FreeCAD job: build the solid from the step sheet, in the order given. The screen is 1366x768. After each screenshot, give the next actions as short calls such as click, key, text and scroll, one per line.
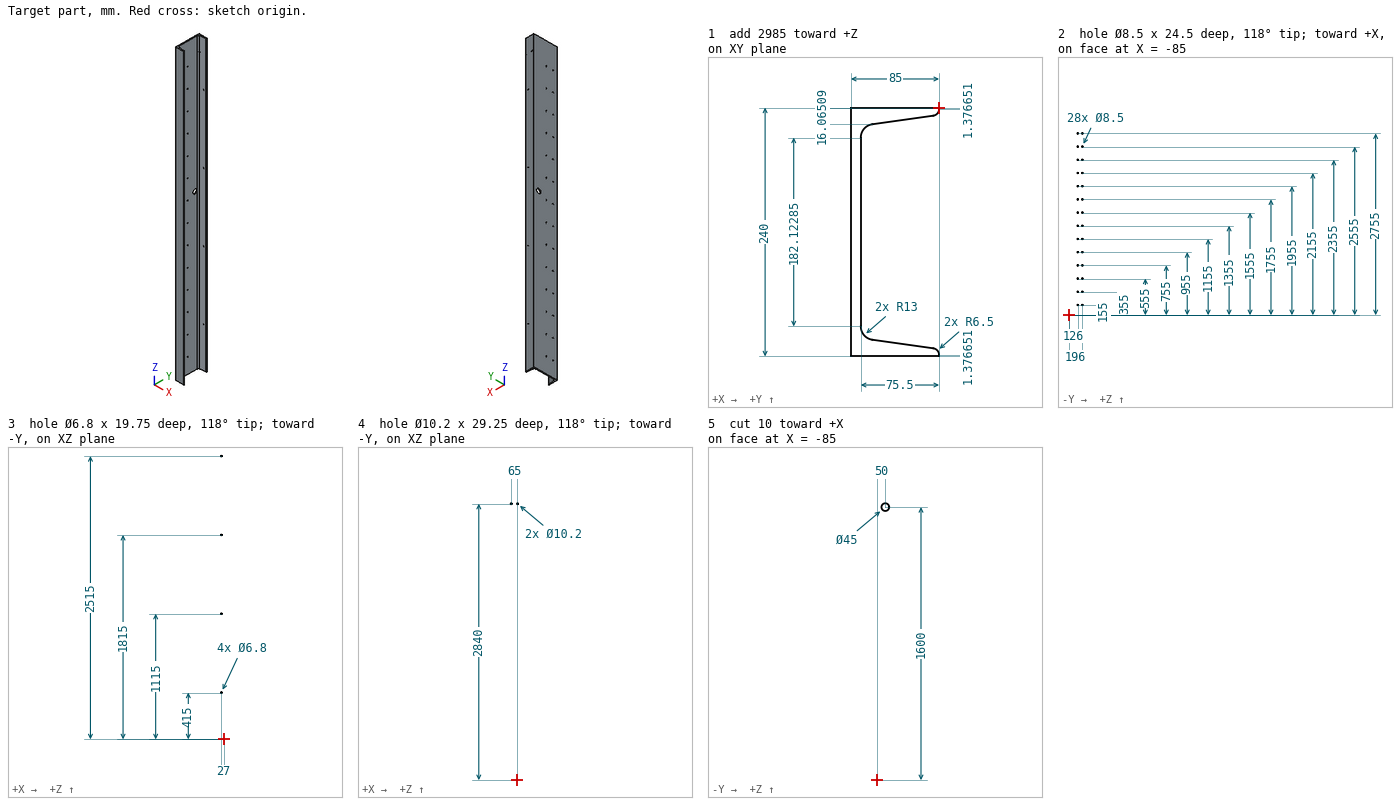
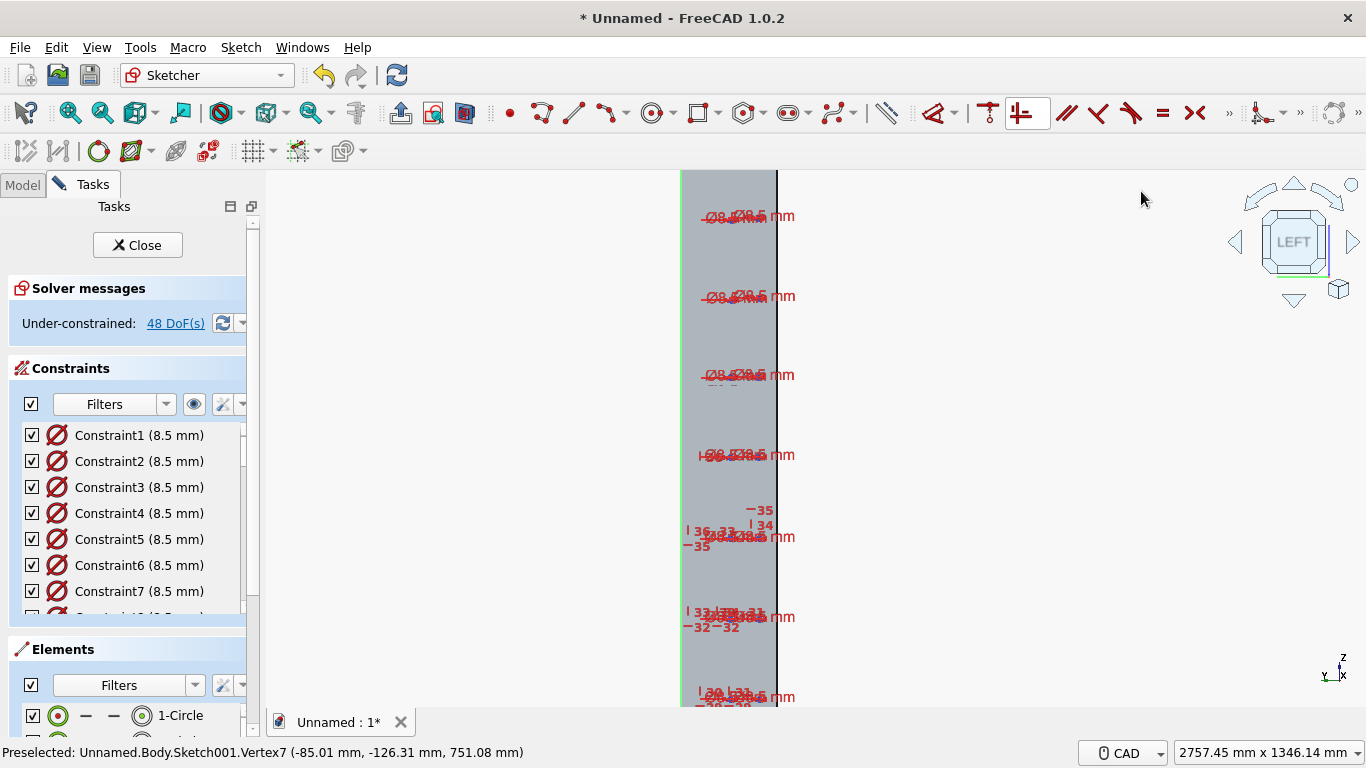
click(759, 539)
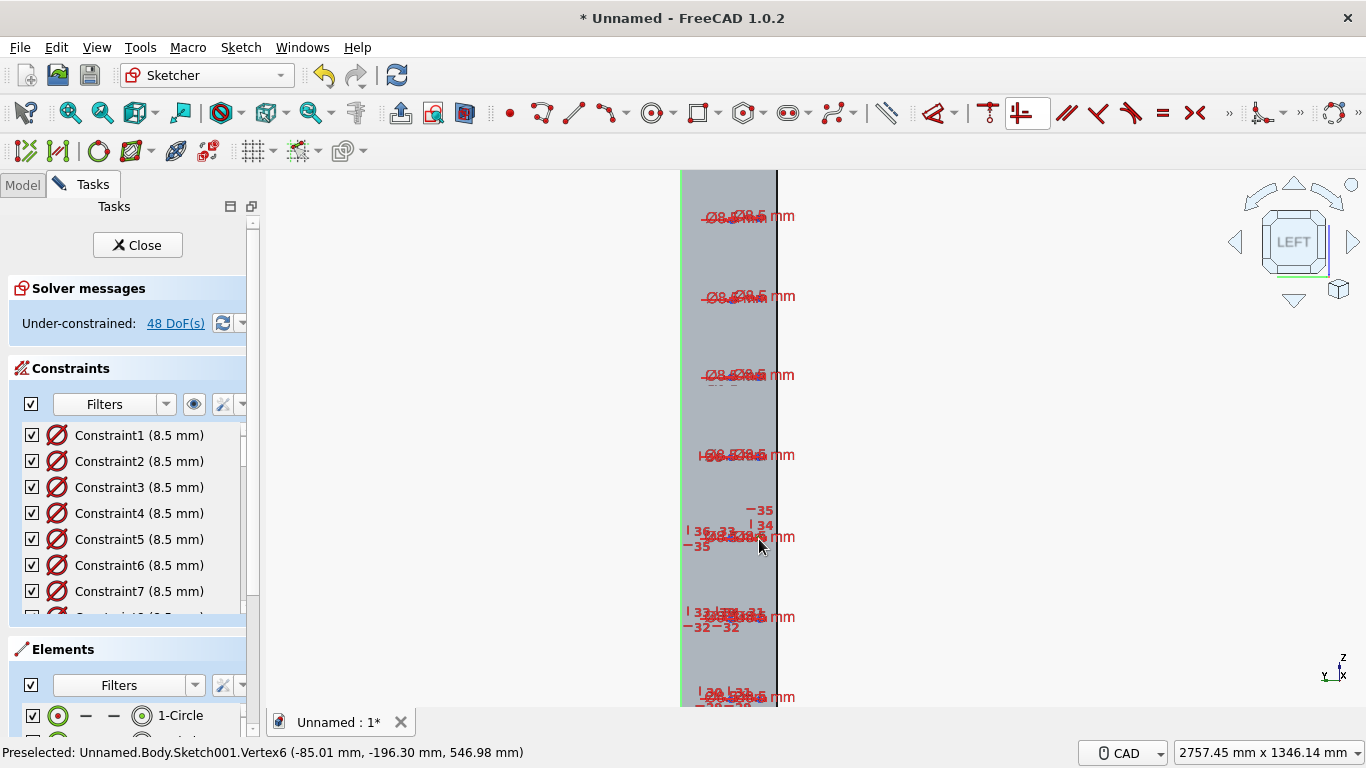
click(759, 457)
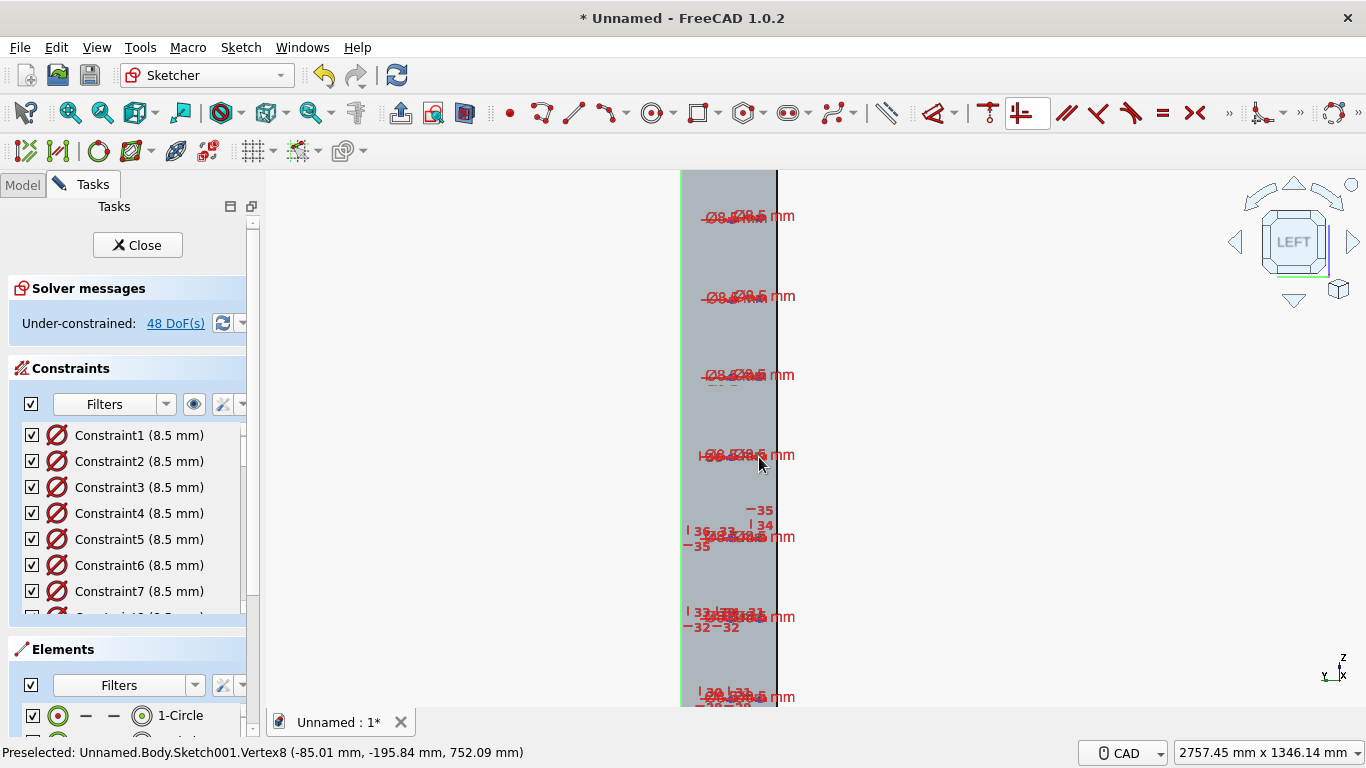
click(1044, 114)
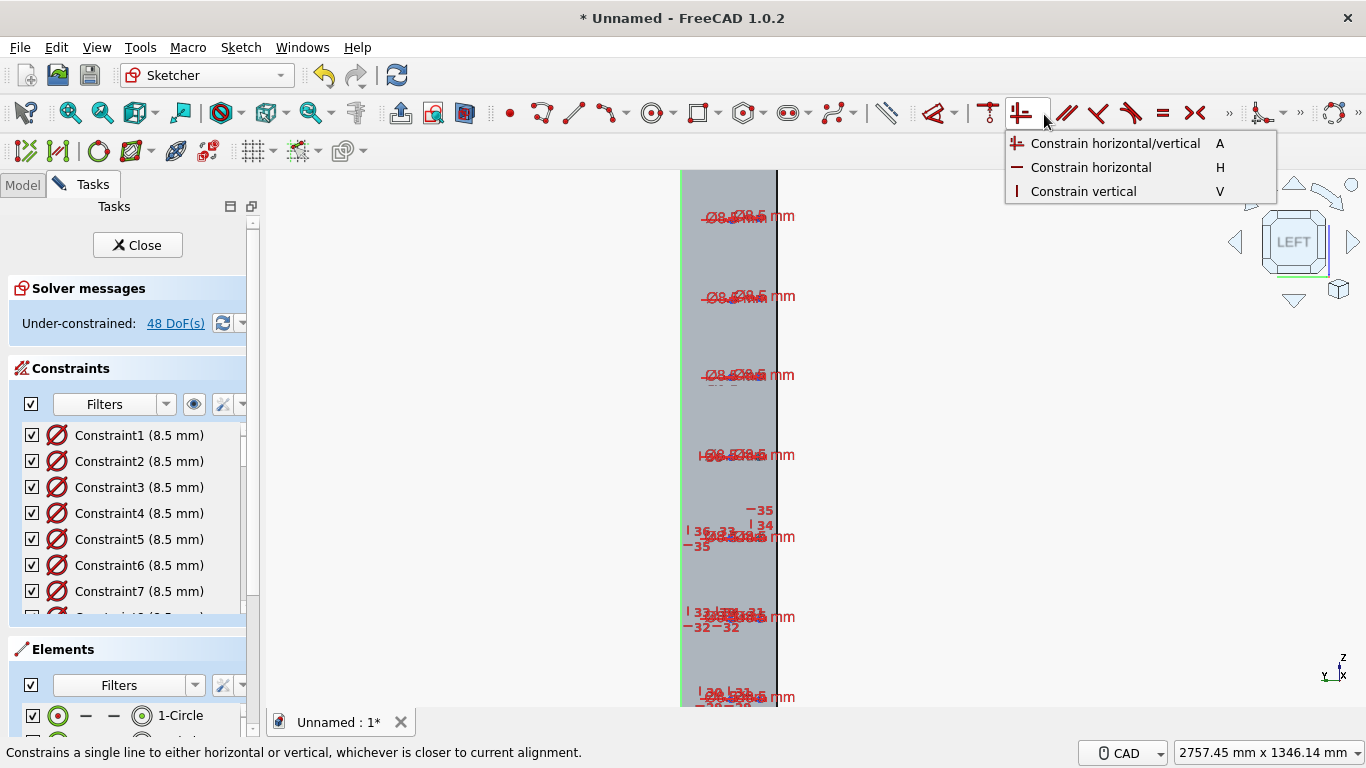
click(1141, 191)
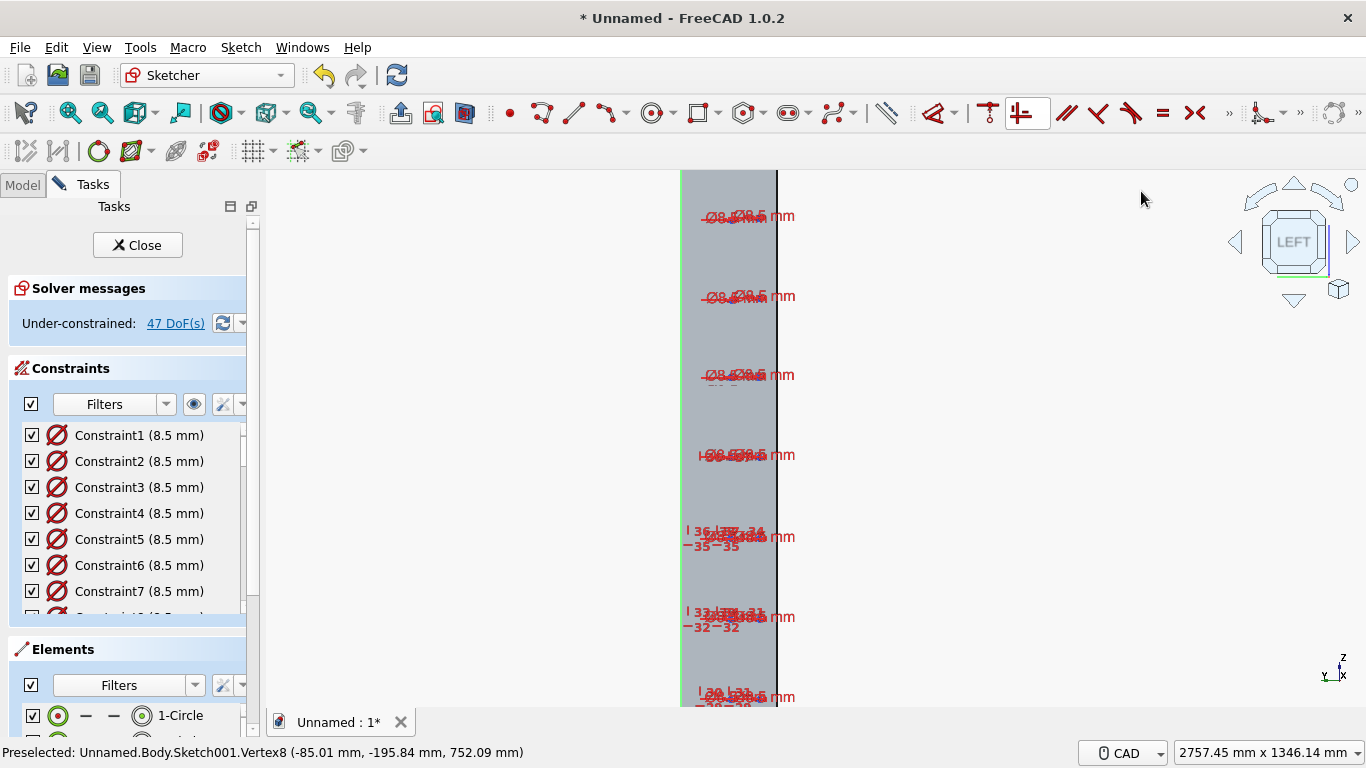
scroll(730, 457, up, 4)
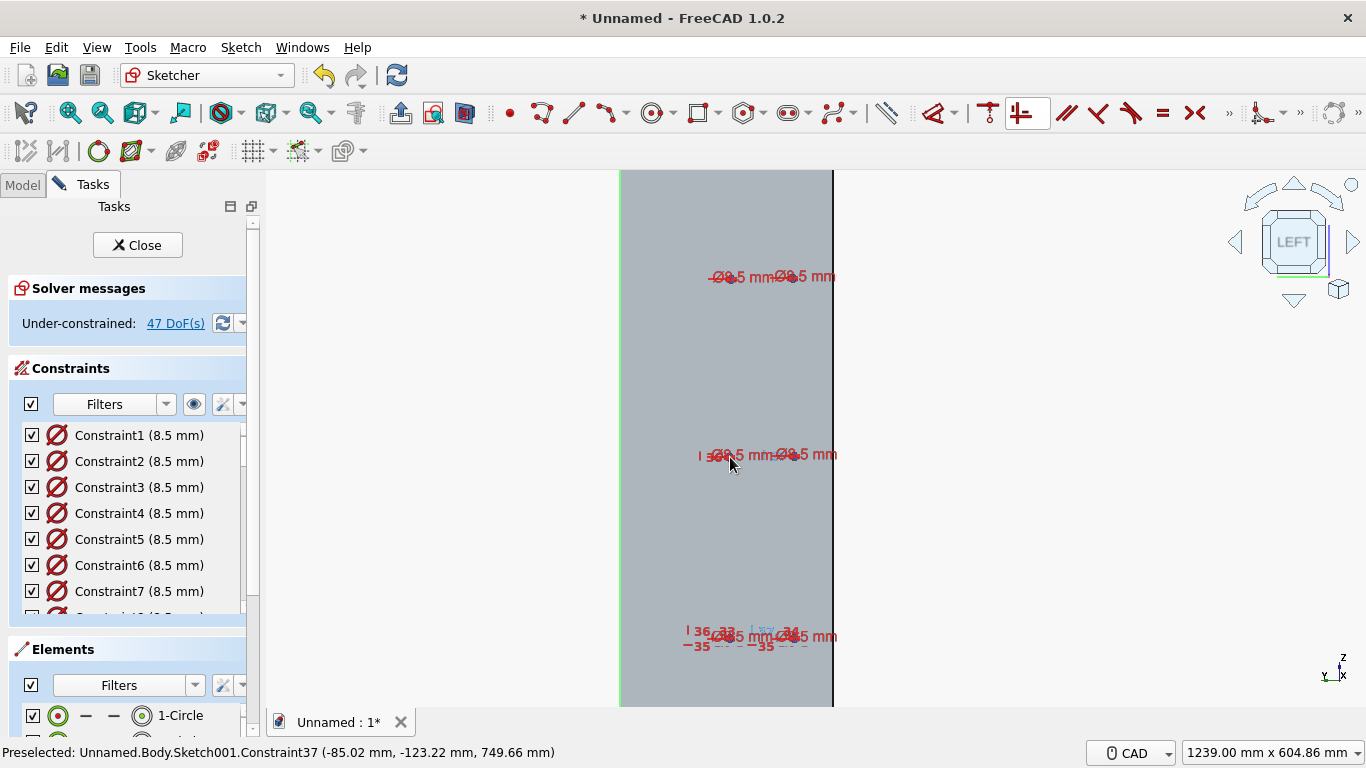
click(730, 457)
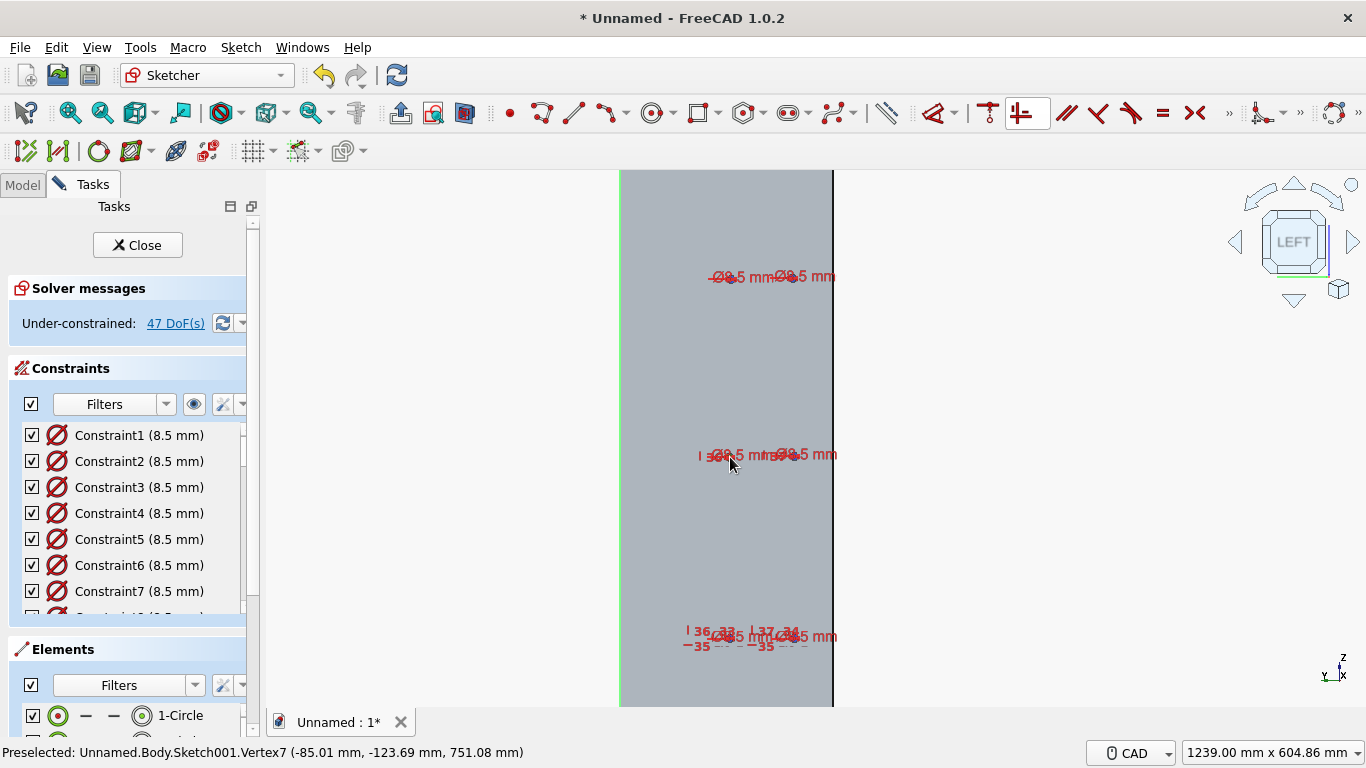
scroll(754, 523, down, 10)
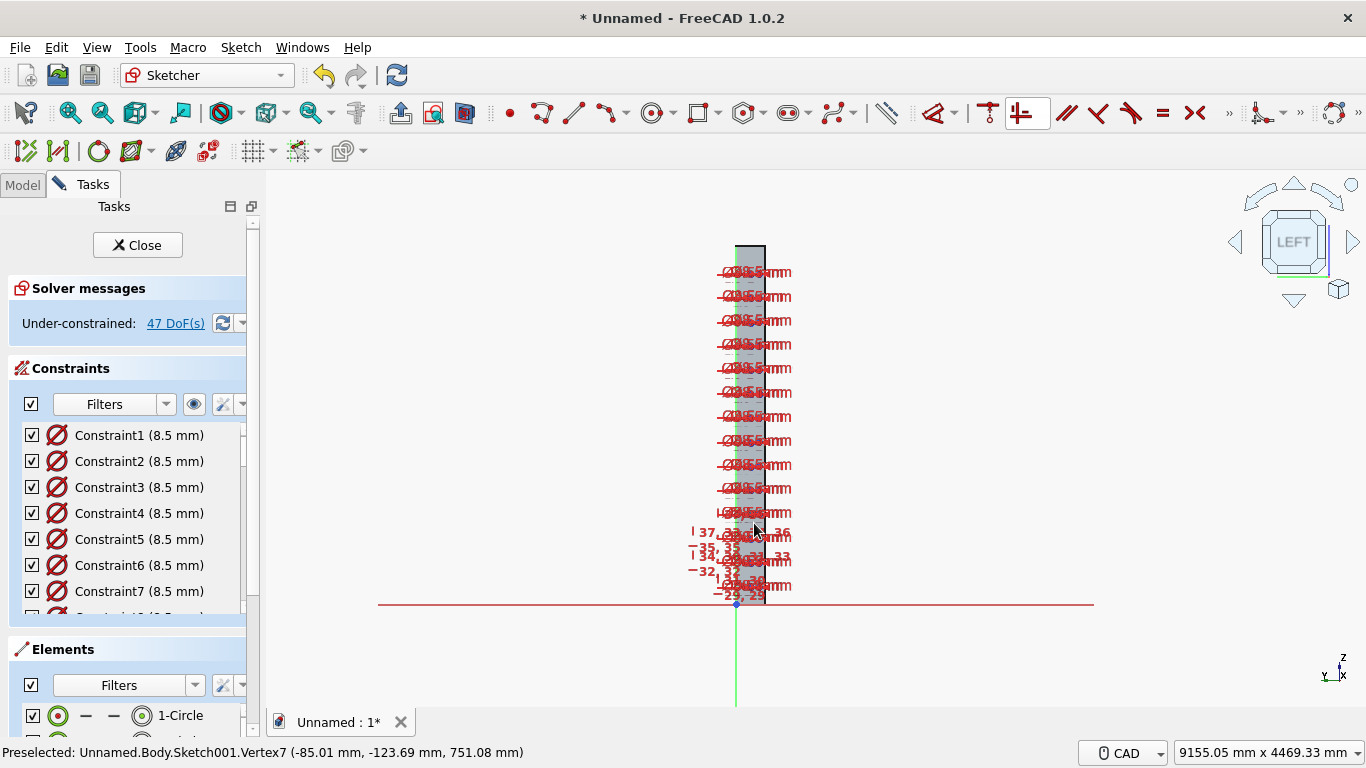
scroll(760, 515, up, 2)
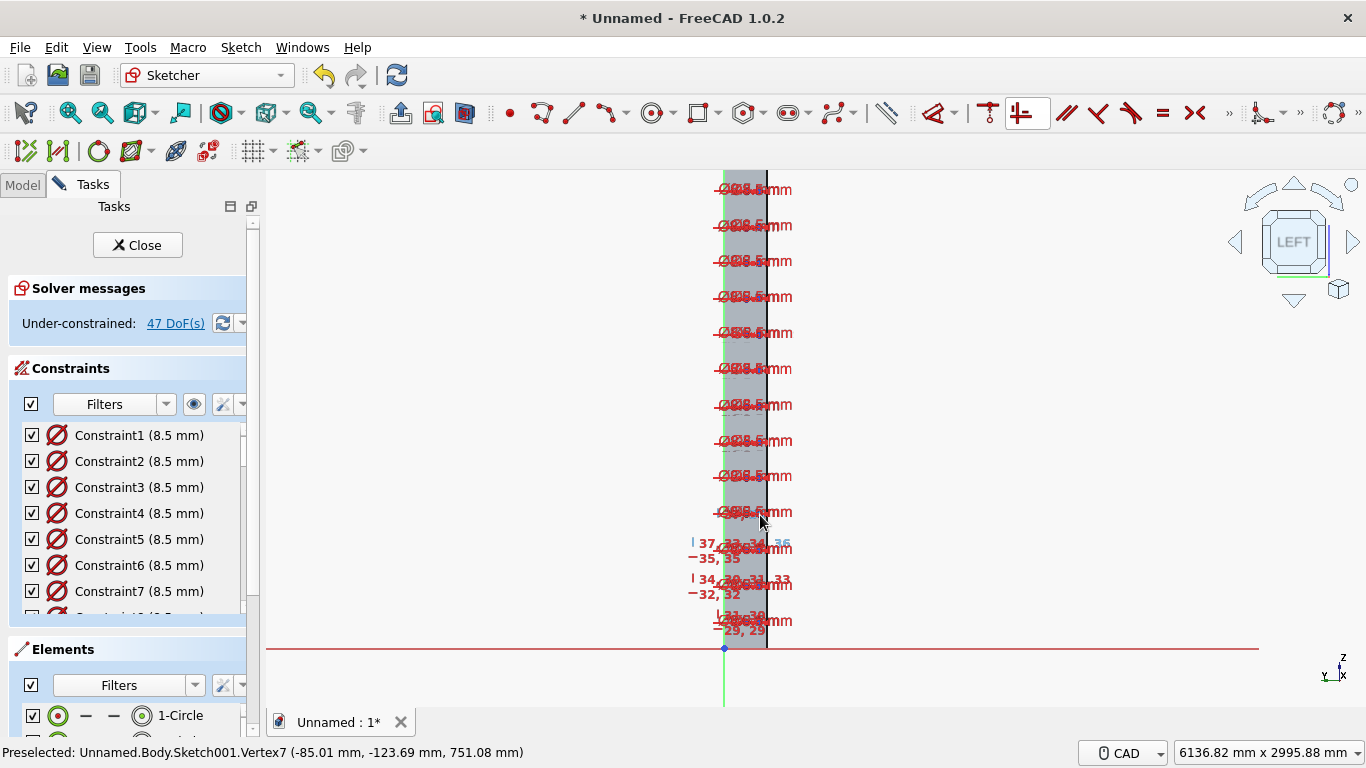
scroll(760, 514, up, 4)